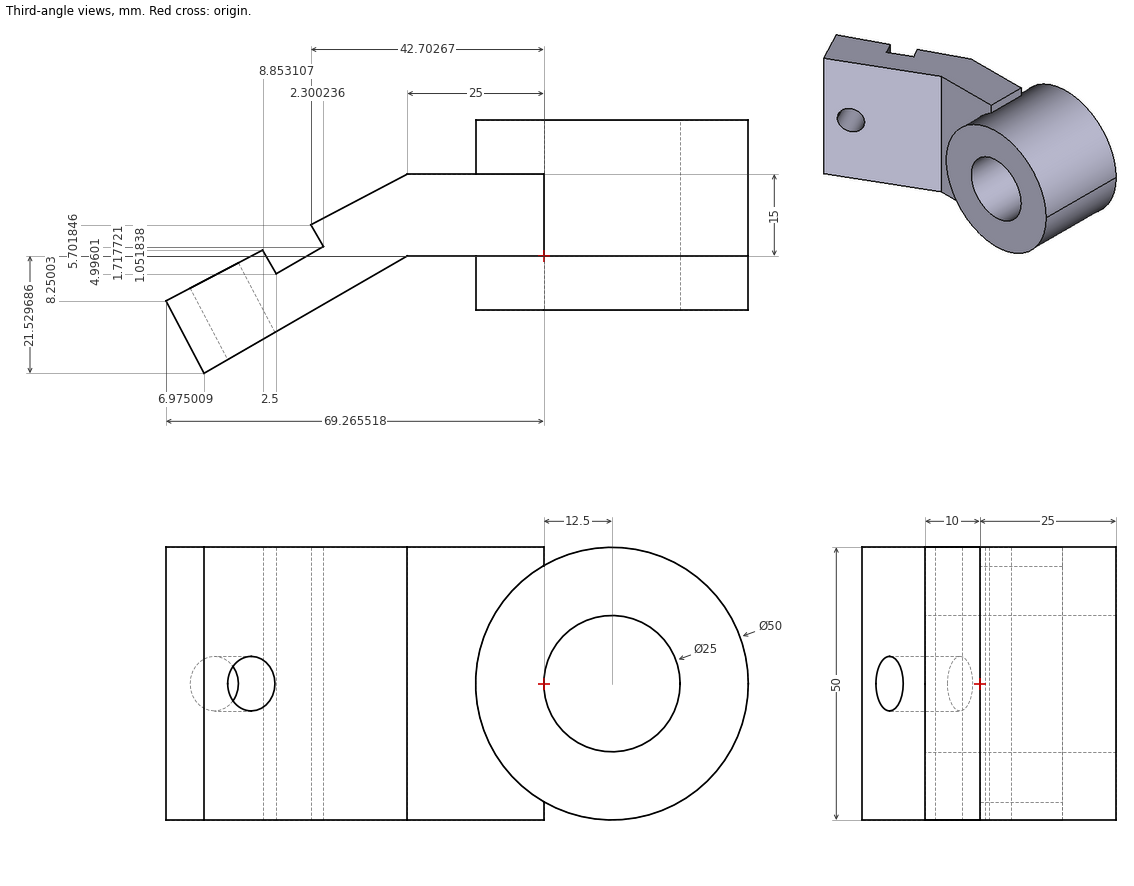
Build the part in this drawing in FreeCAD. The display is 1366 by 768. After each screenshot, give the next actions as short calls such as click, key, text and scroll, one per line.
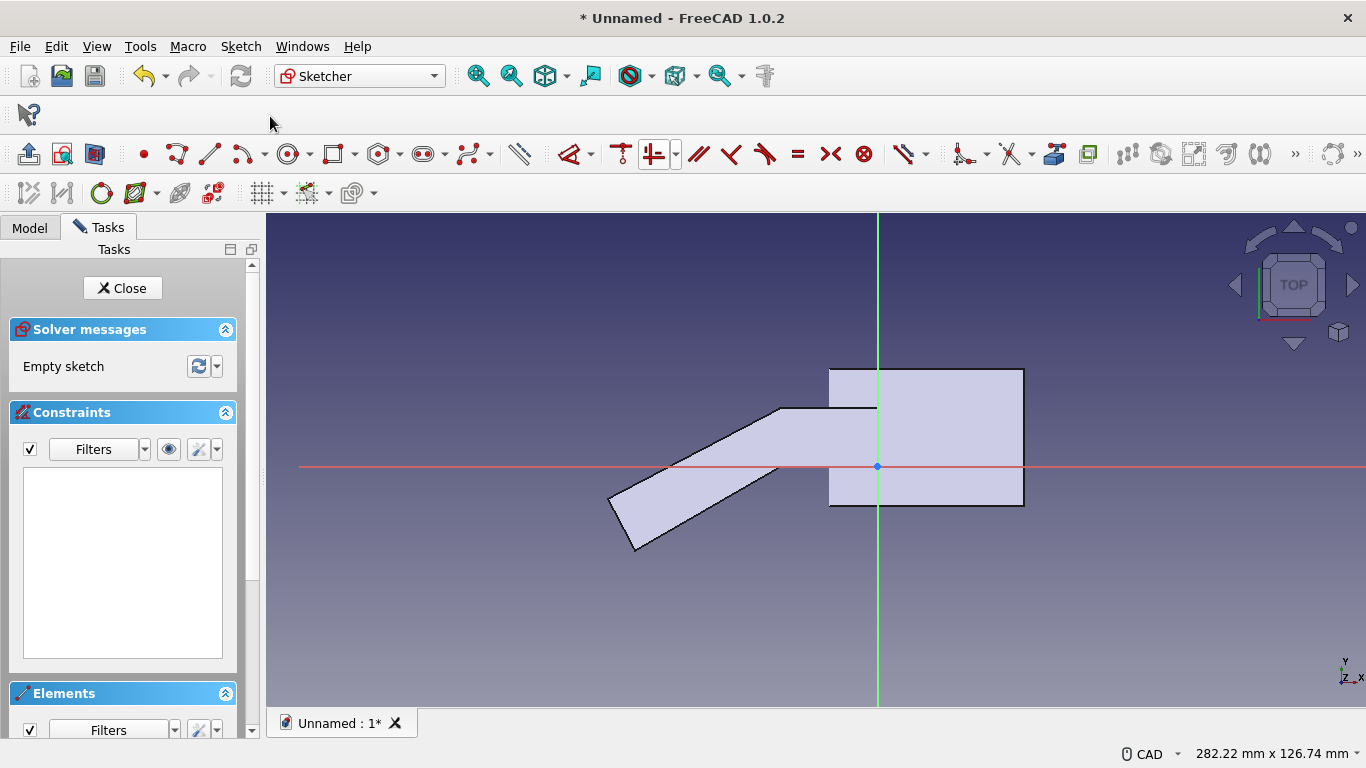
scroll(693, 462, up, 11)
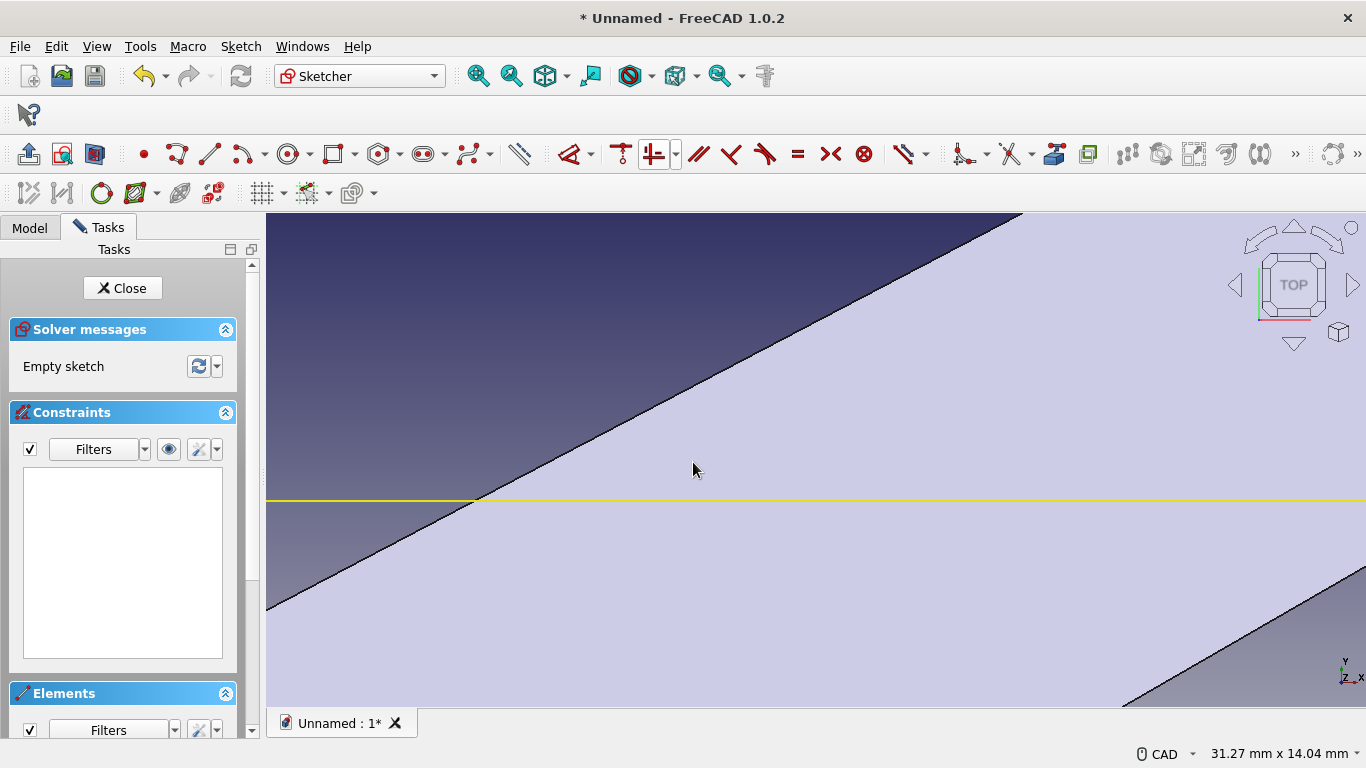
key(g)
key(m)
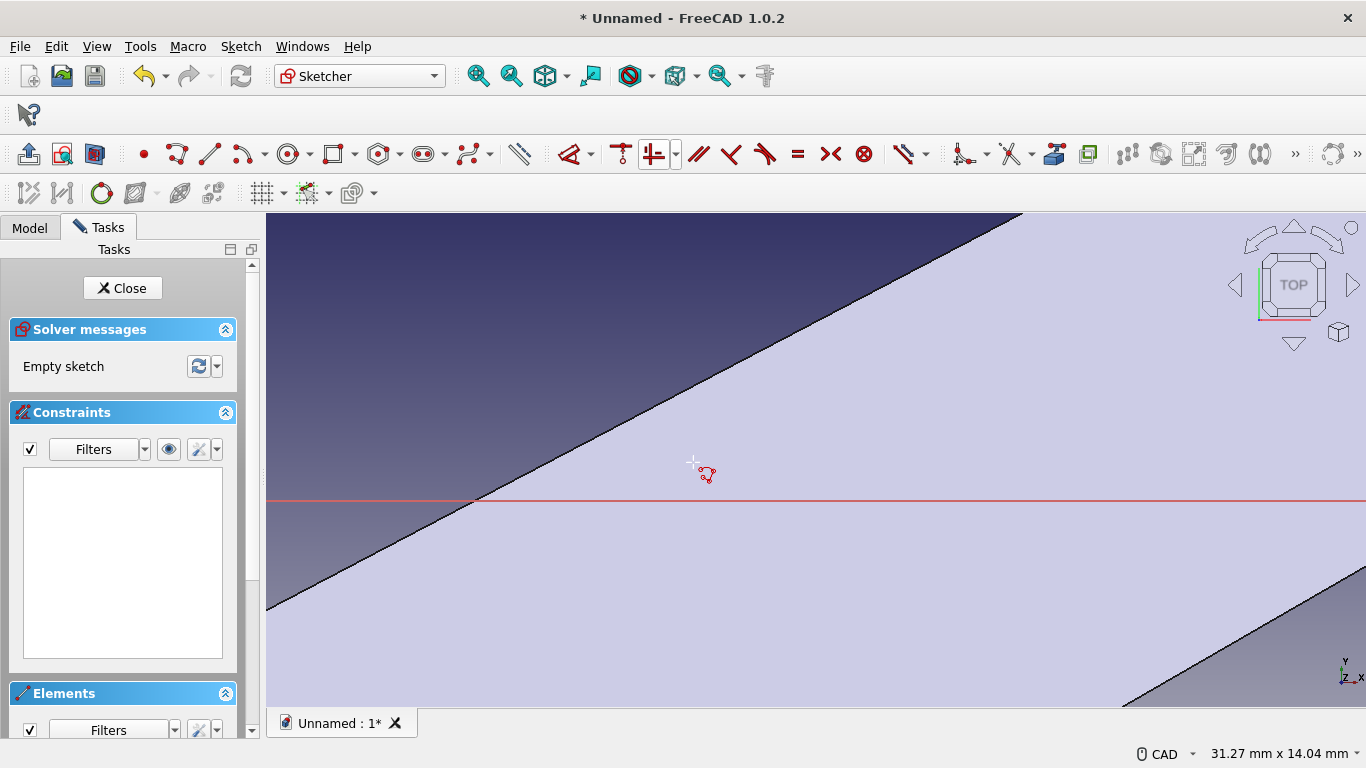
click(937, 441)
click(857, 300)
click(545, 464)
click(633, 616)
click(937, 442)
key(Escape)
key(Escape)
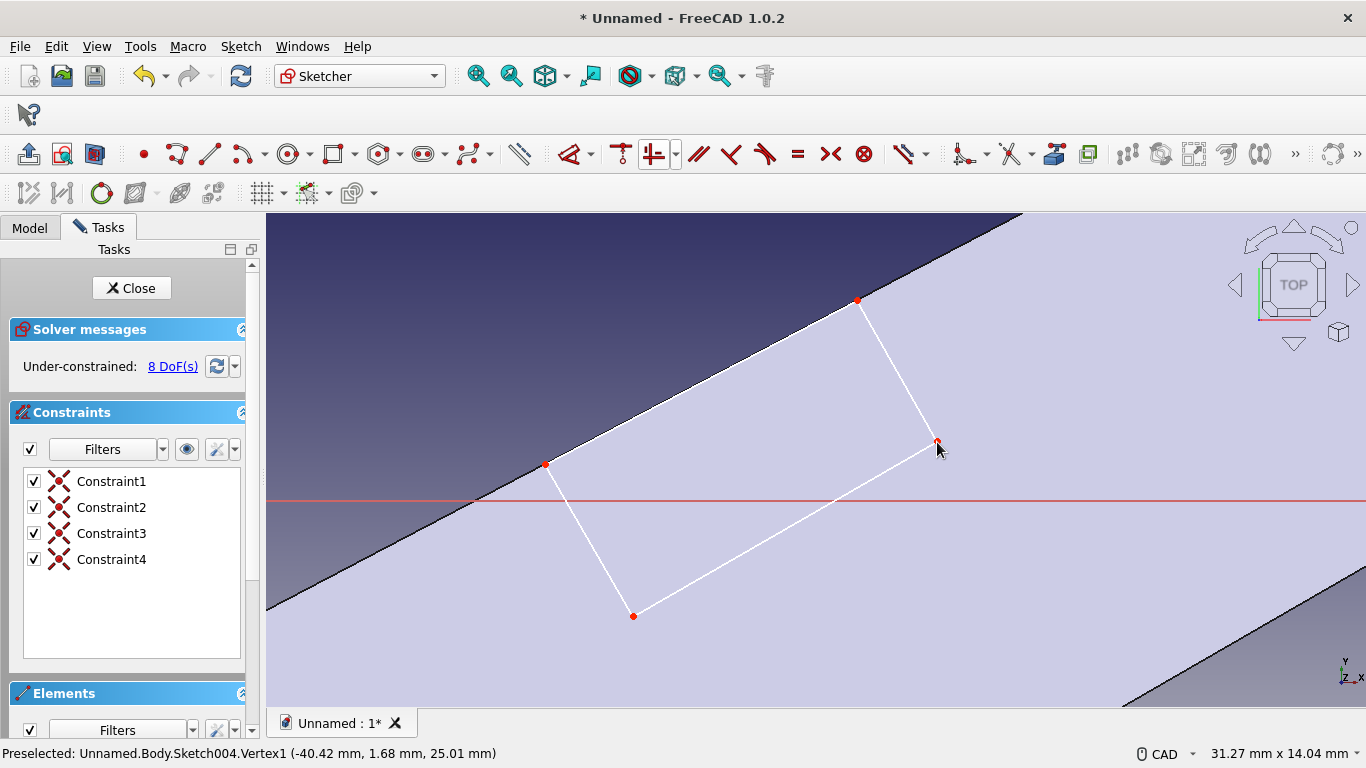
key(d)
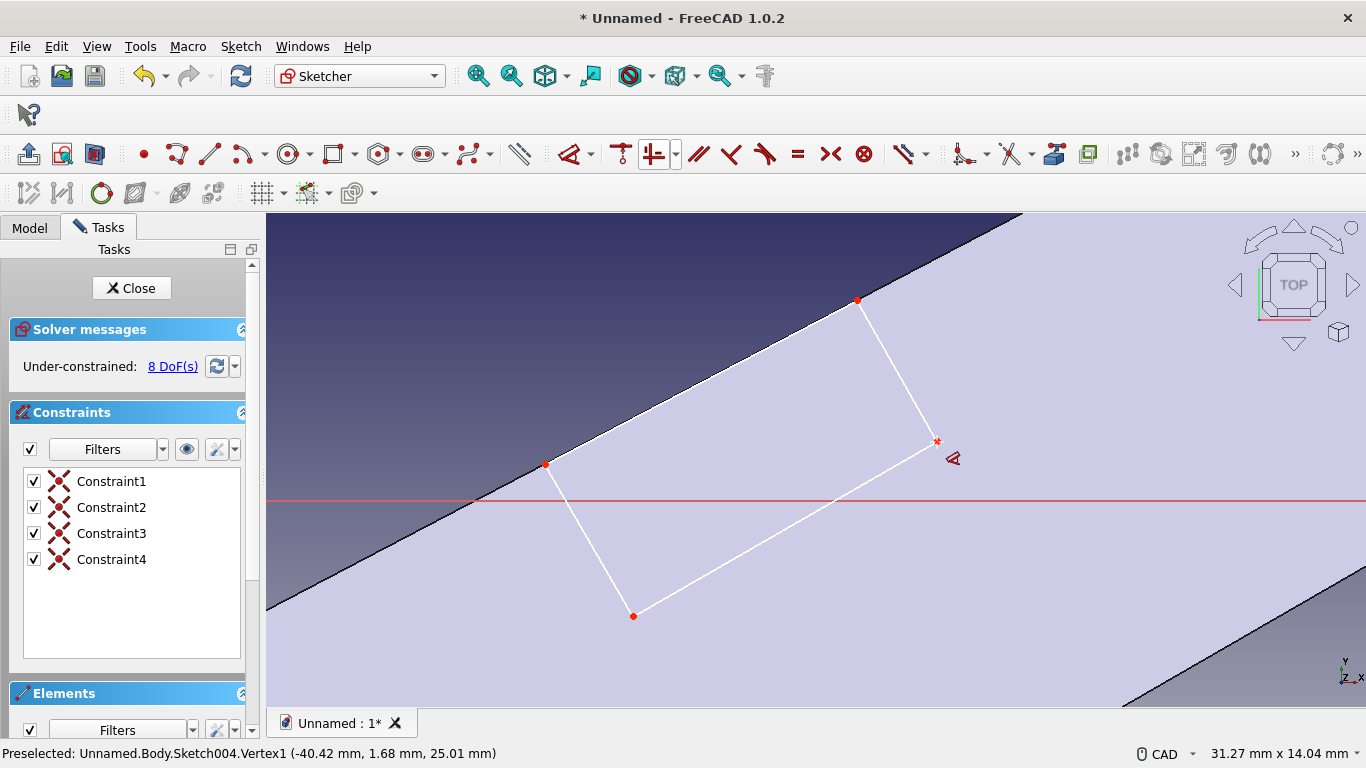
scroll(571, 511, up, 2)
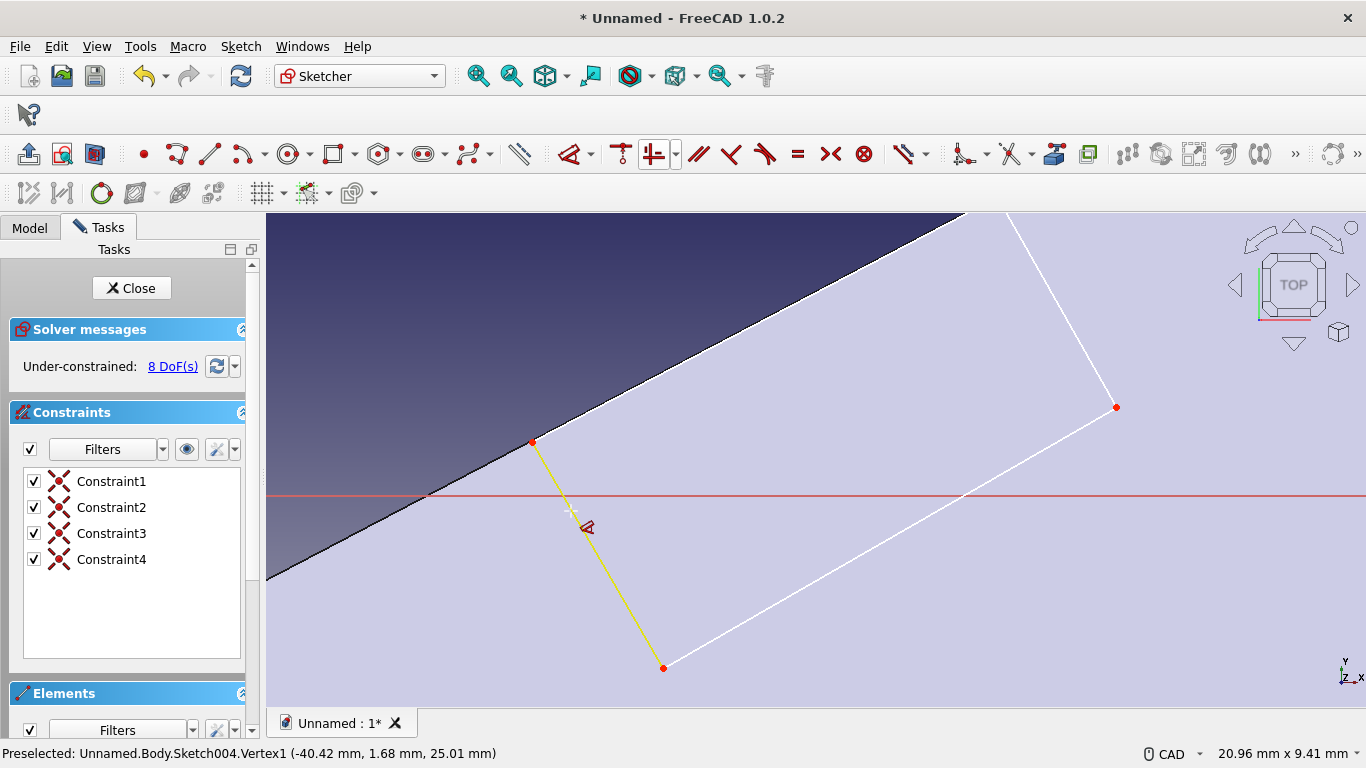
click(571, 510)
click(568, 408)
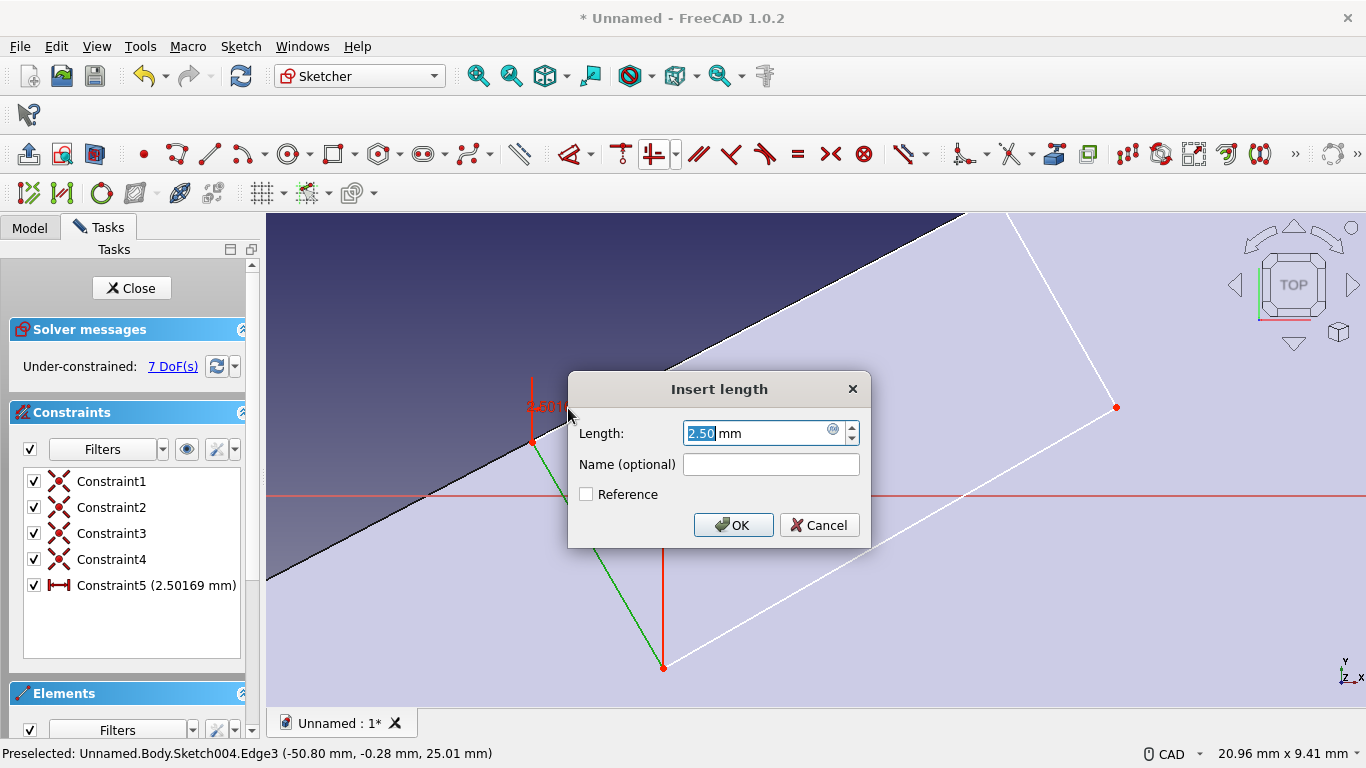
text(2.5)
key(Return)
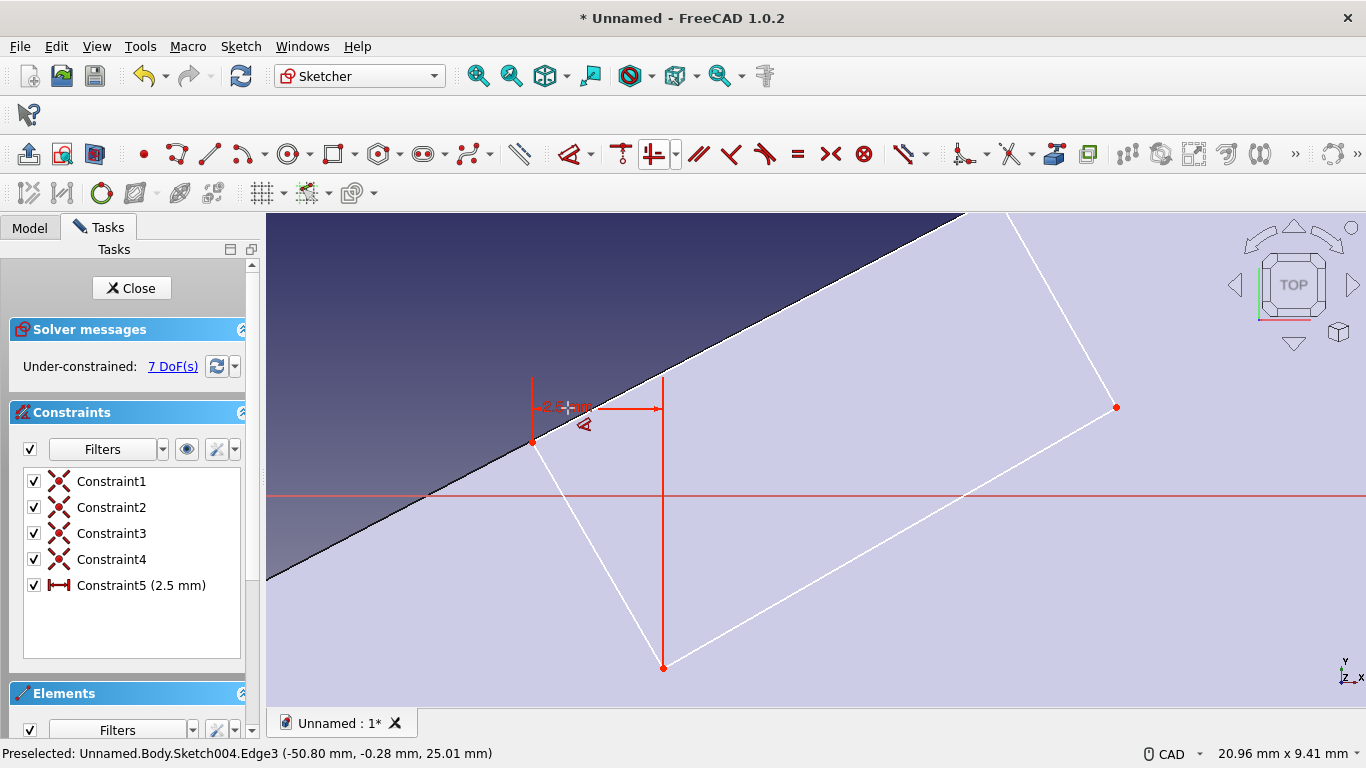
click(799, 591)
click(1151, 538)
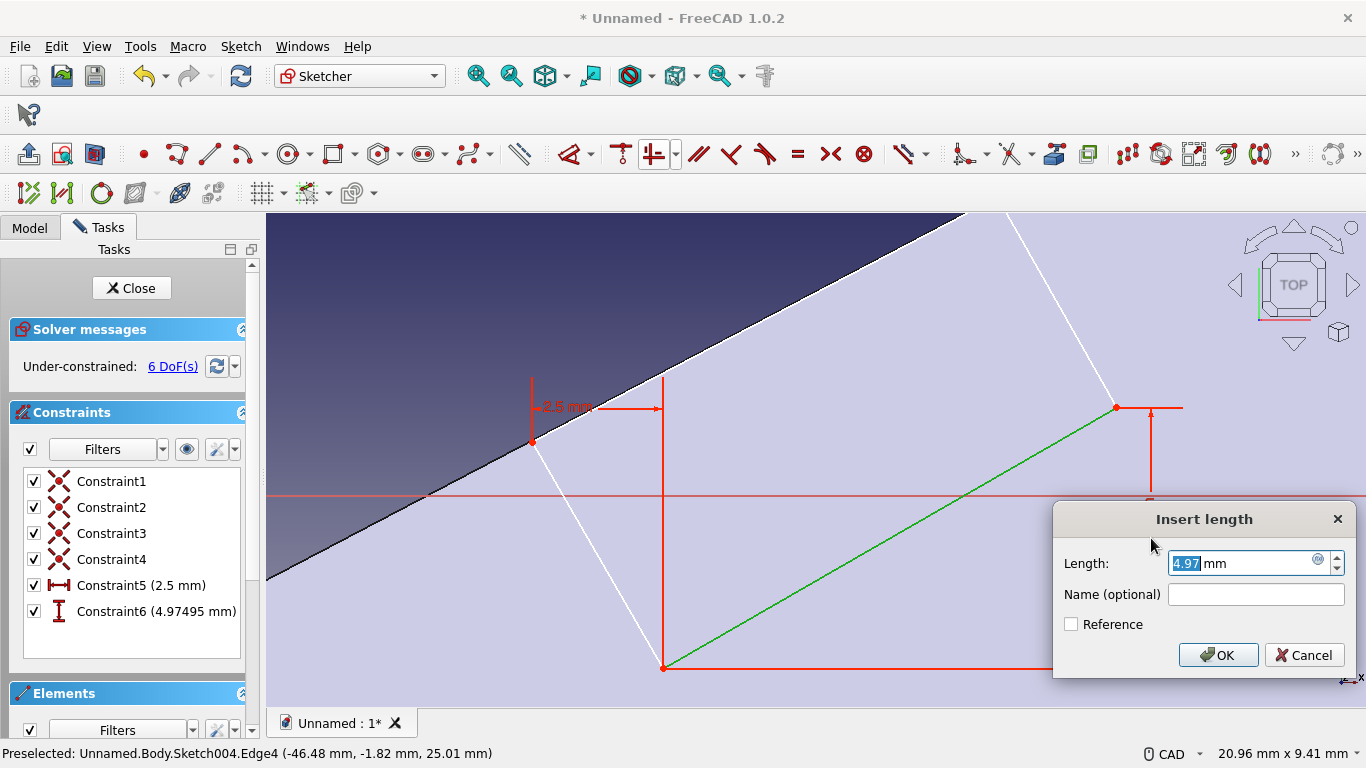
text(4.99601)
key(Return)